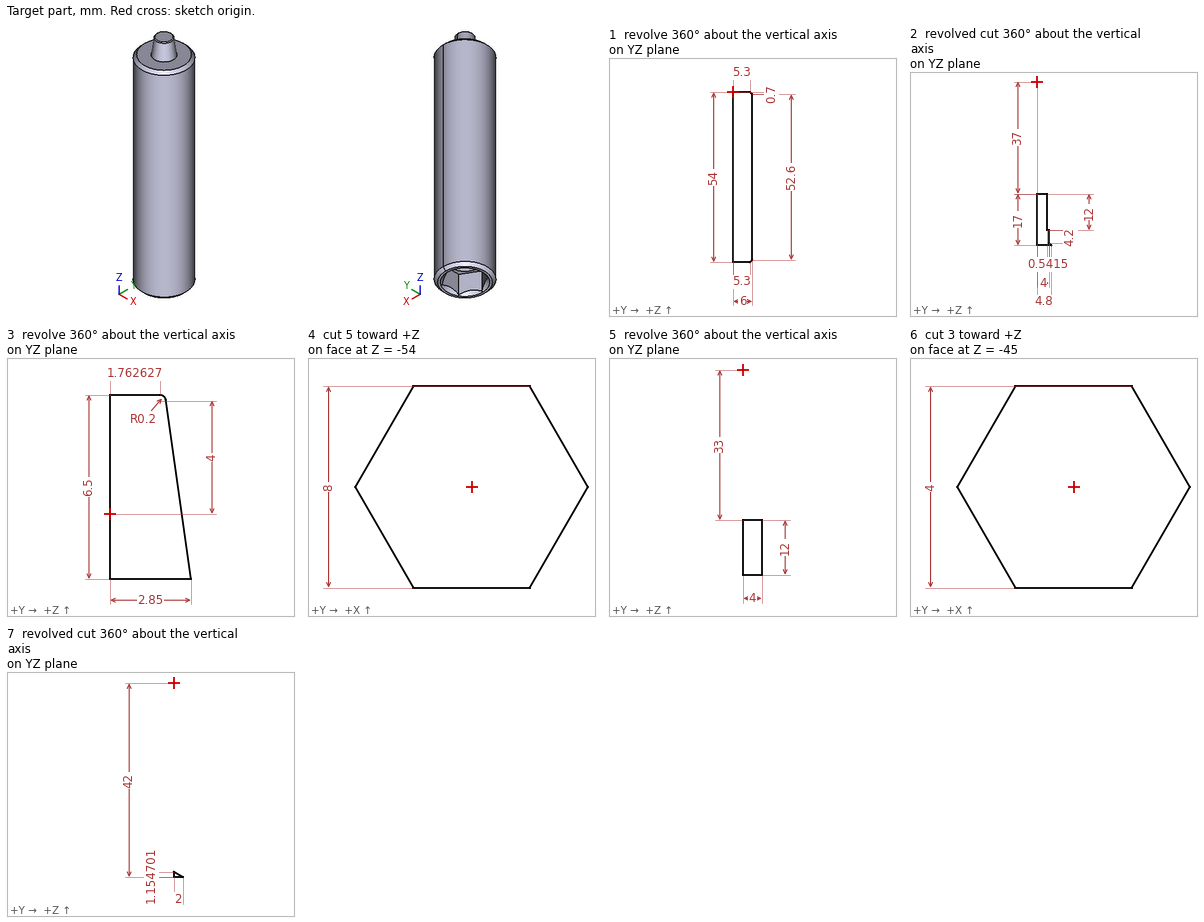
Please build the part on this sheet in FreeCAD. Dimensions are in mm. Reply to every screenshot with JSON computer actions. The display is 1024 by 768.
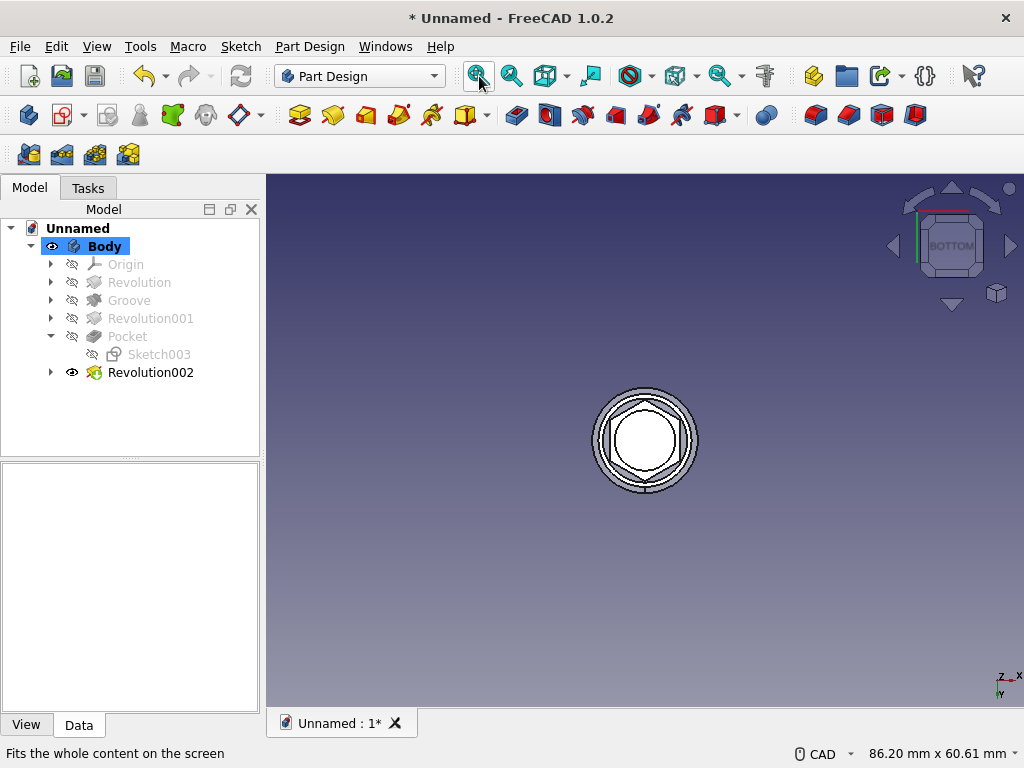
{"action": "left_click", "coordinate": [645, 439]}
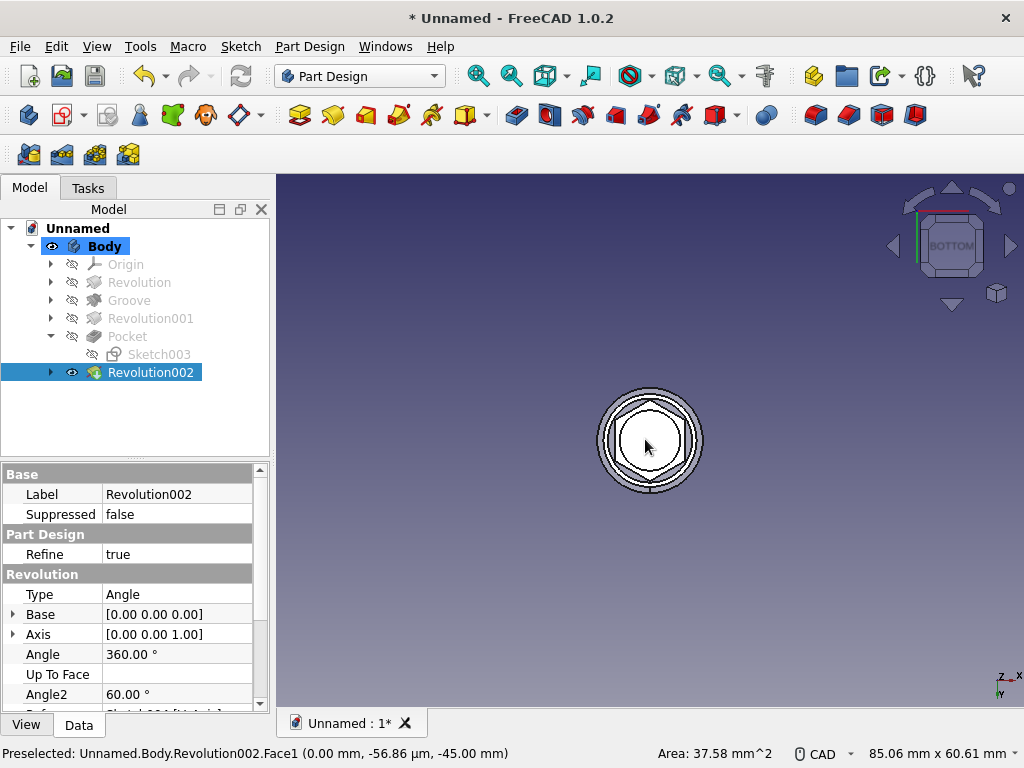
{"action": "left_click", "coordinate": [62, 116]}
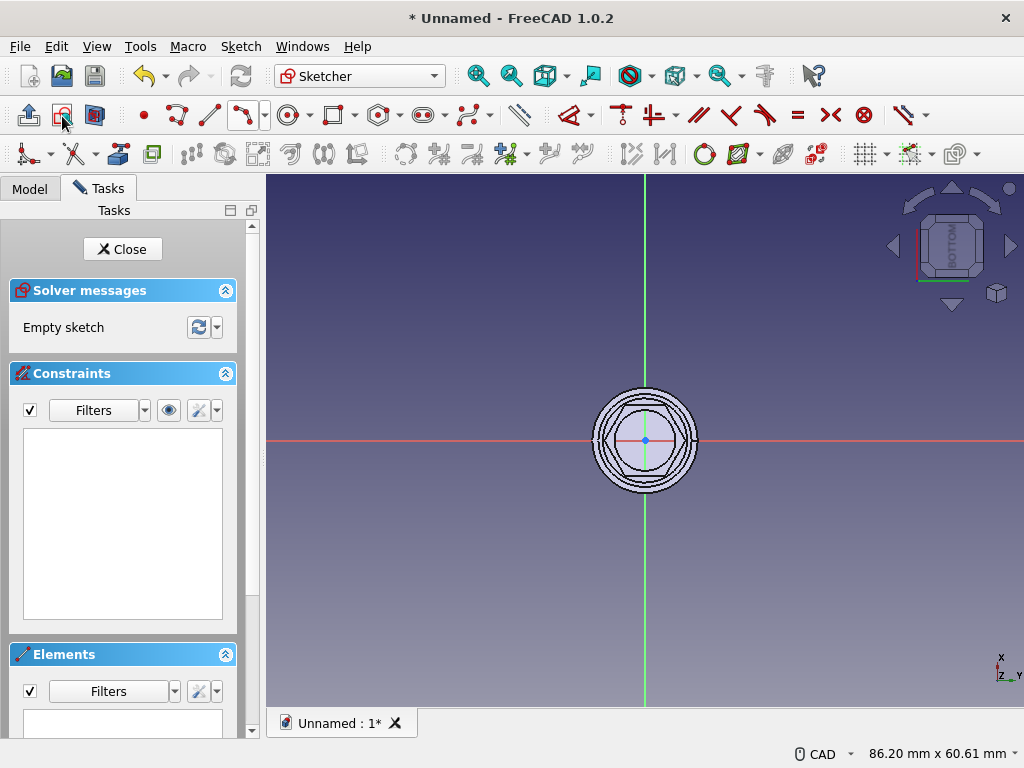
{"action": "scroll", "coordinate": [654, 440], "scroll_direction": "up", "scroll_amount": 11}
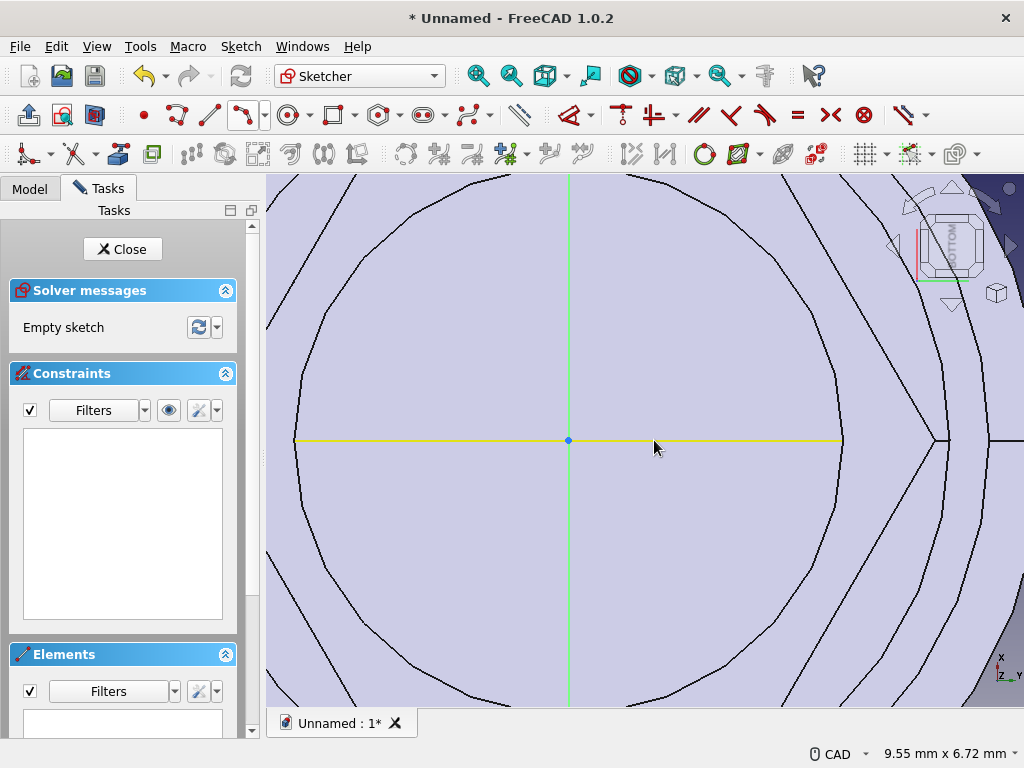
{"action": "left_click", "coordinate": [378, 116]}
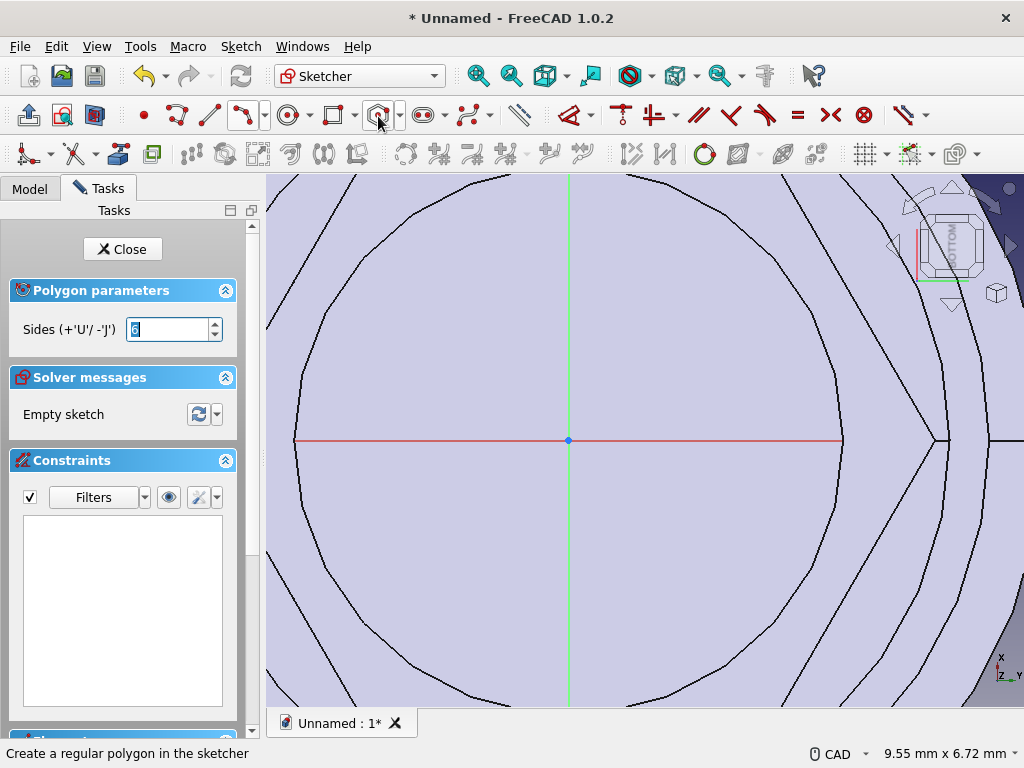
{"action": "left_click", "coordinate": [569, 440]}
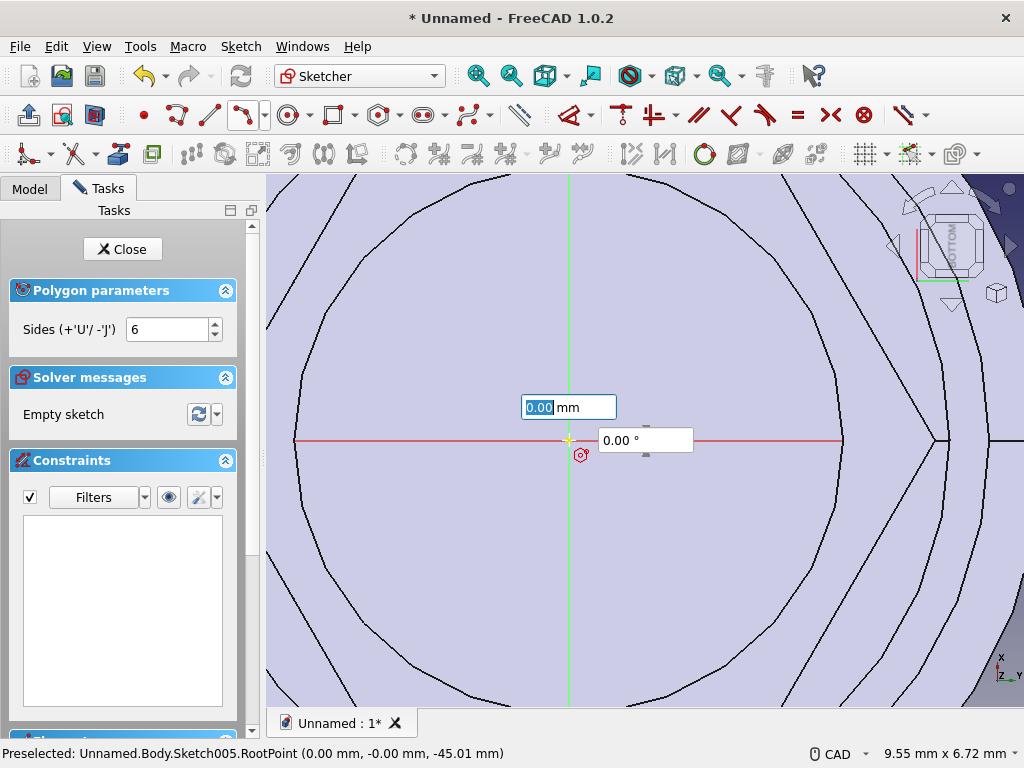
{"action": "left_click", "coordinate": [385, 440]}
{"action": "right_click", "coordinate": [385, 440]}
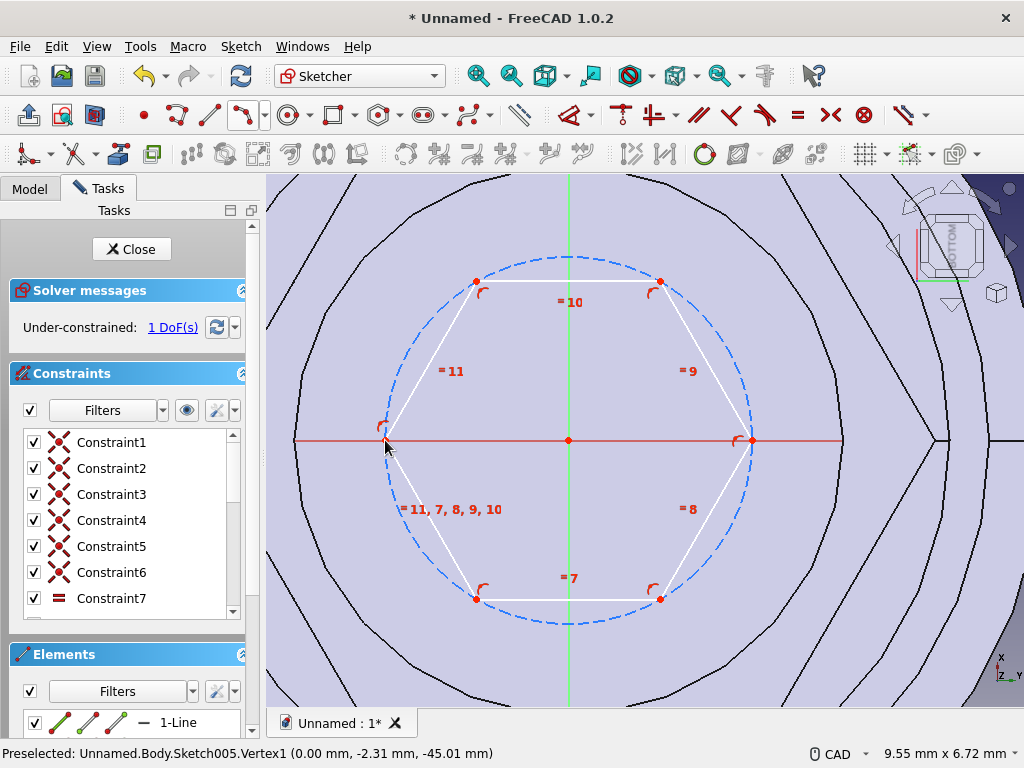
{"action": "left_click", "coordinate": [568, 116]}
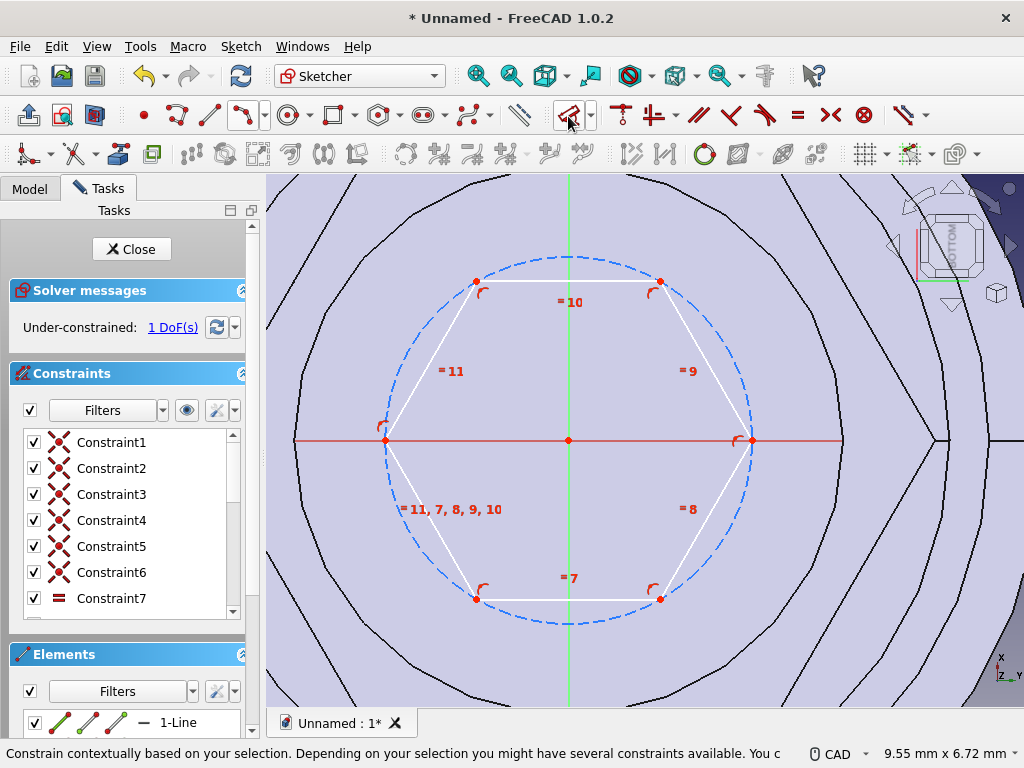
{"action": "left_click", "coordinate": [477, 600]}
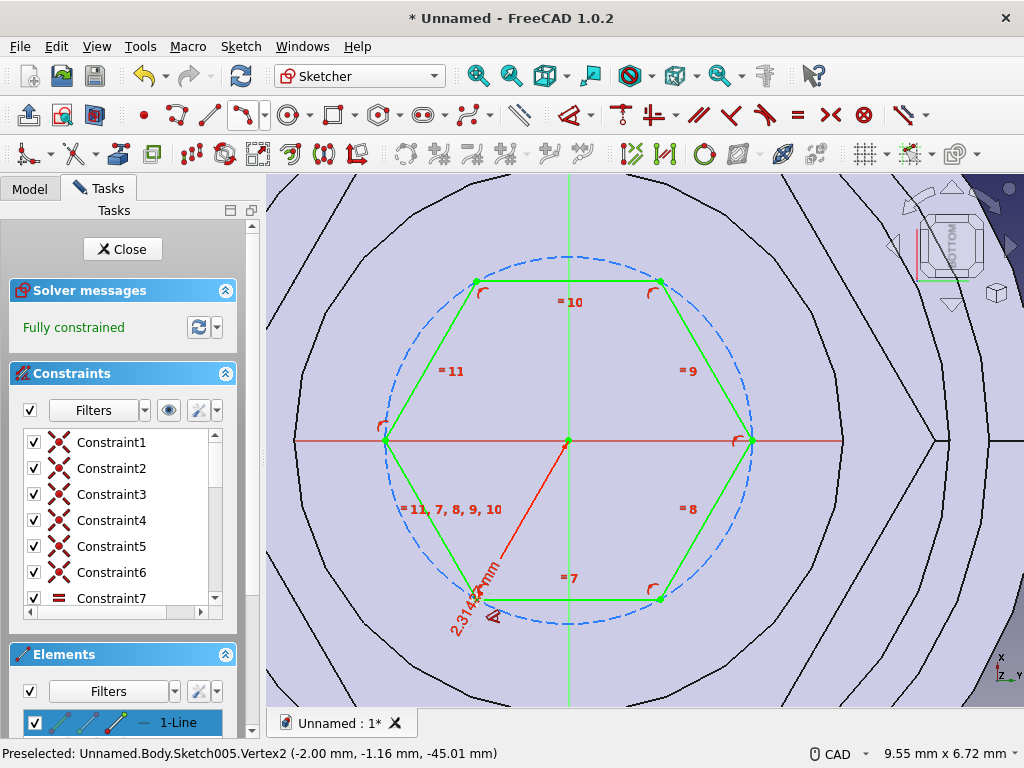
{"action": "left_click", "coordinate": [660, 281]}
{"action": "left_click", "coordinate": [694, 367]}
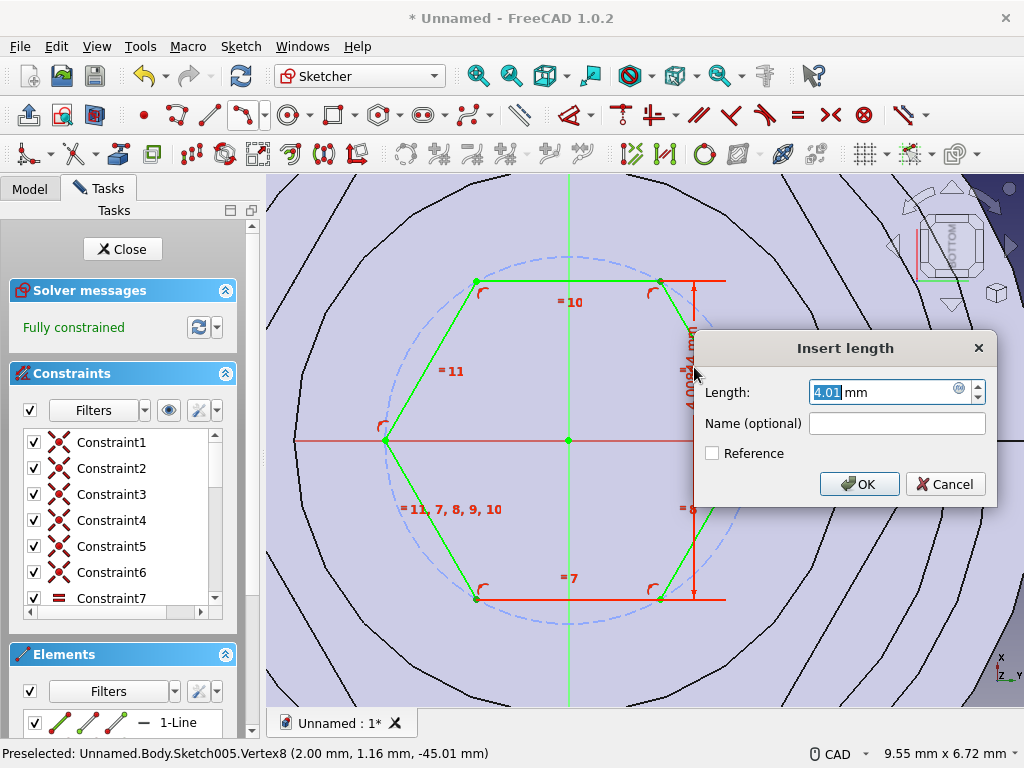
{"action": "type", "text": "4"}
{"action": "key", "text": "Return"}
{"action": "key", "text": "Escape"}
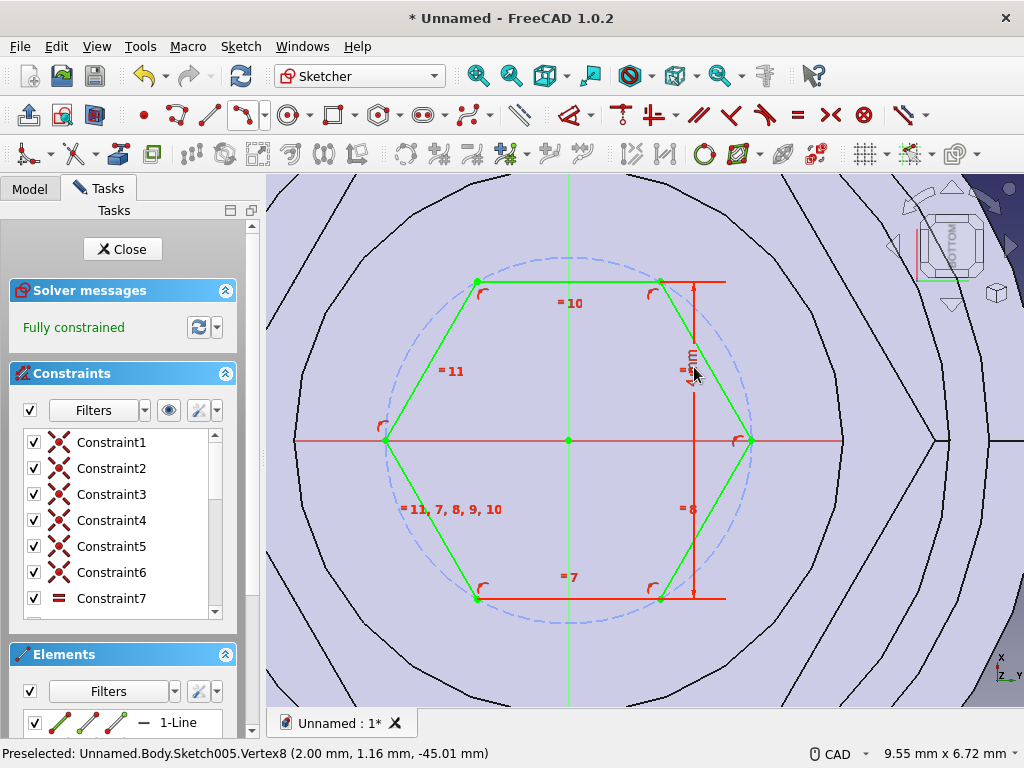
{"action": "left_click", "coordinate": [123, 249]}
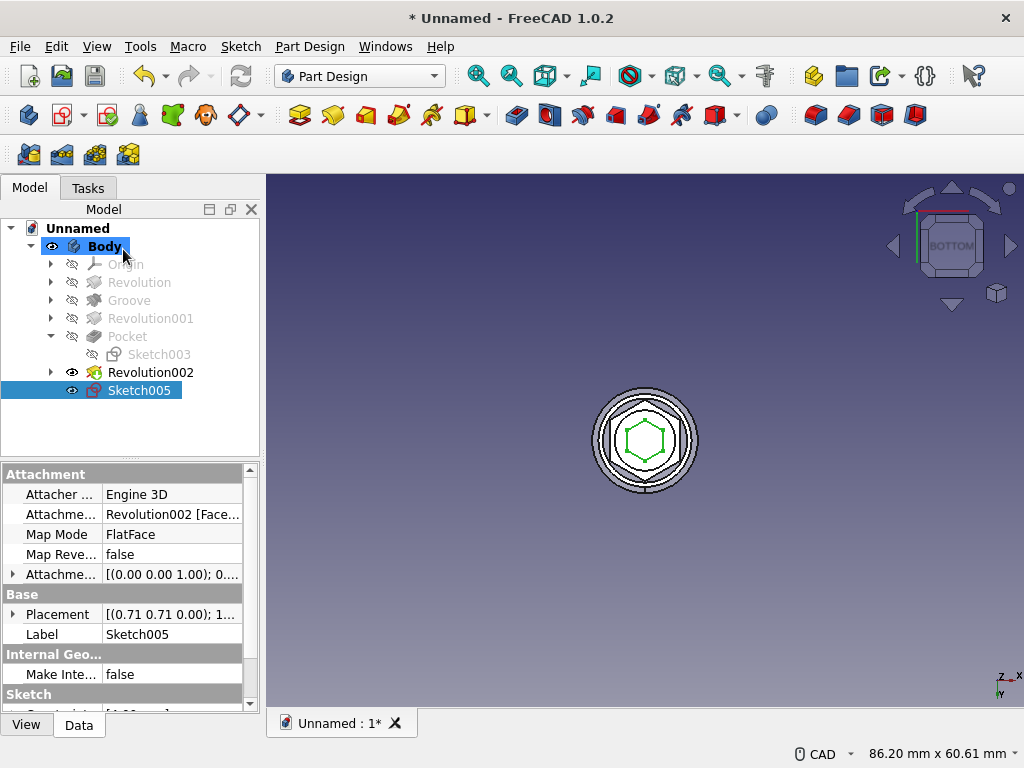
{"action": "left_click", "coordinate": [517, 116]}